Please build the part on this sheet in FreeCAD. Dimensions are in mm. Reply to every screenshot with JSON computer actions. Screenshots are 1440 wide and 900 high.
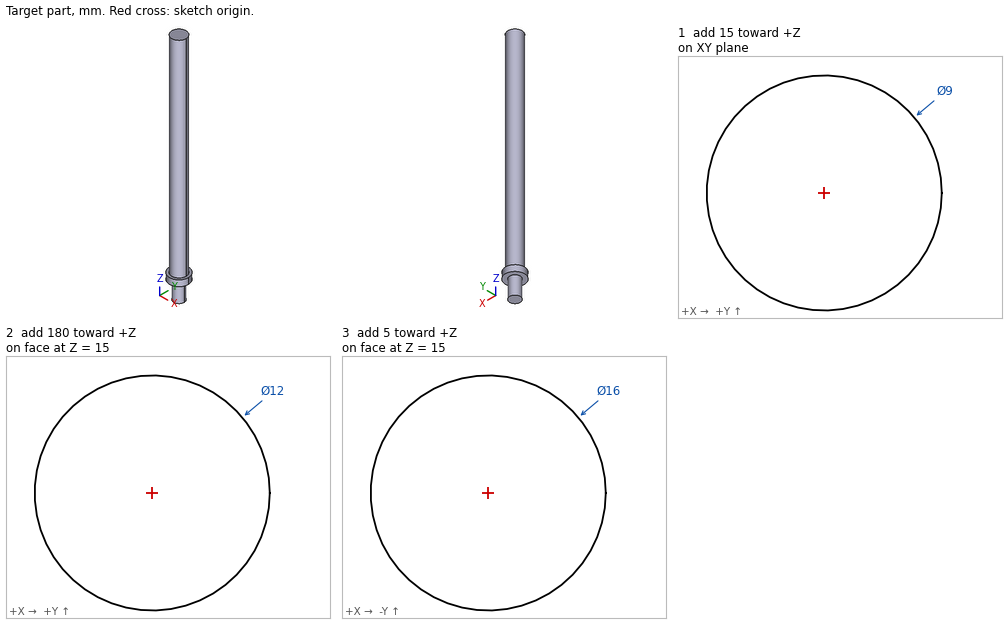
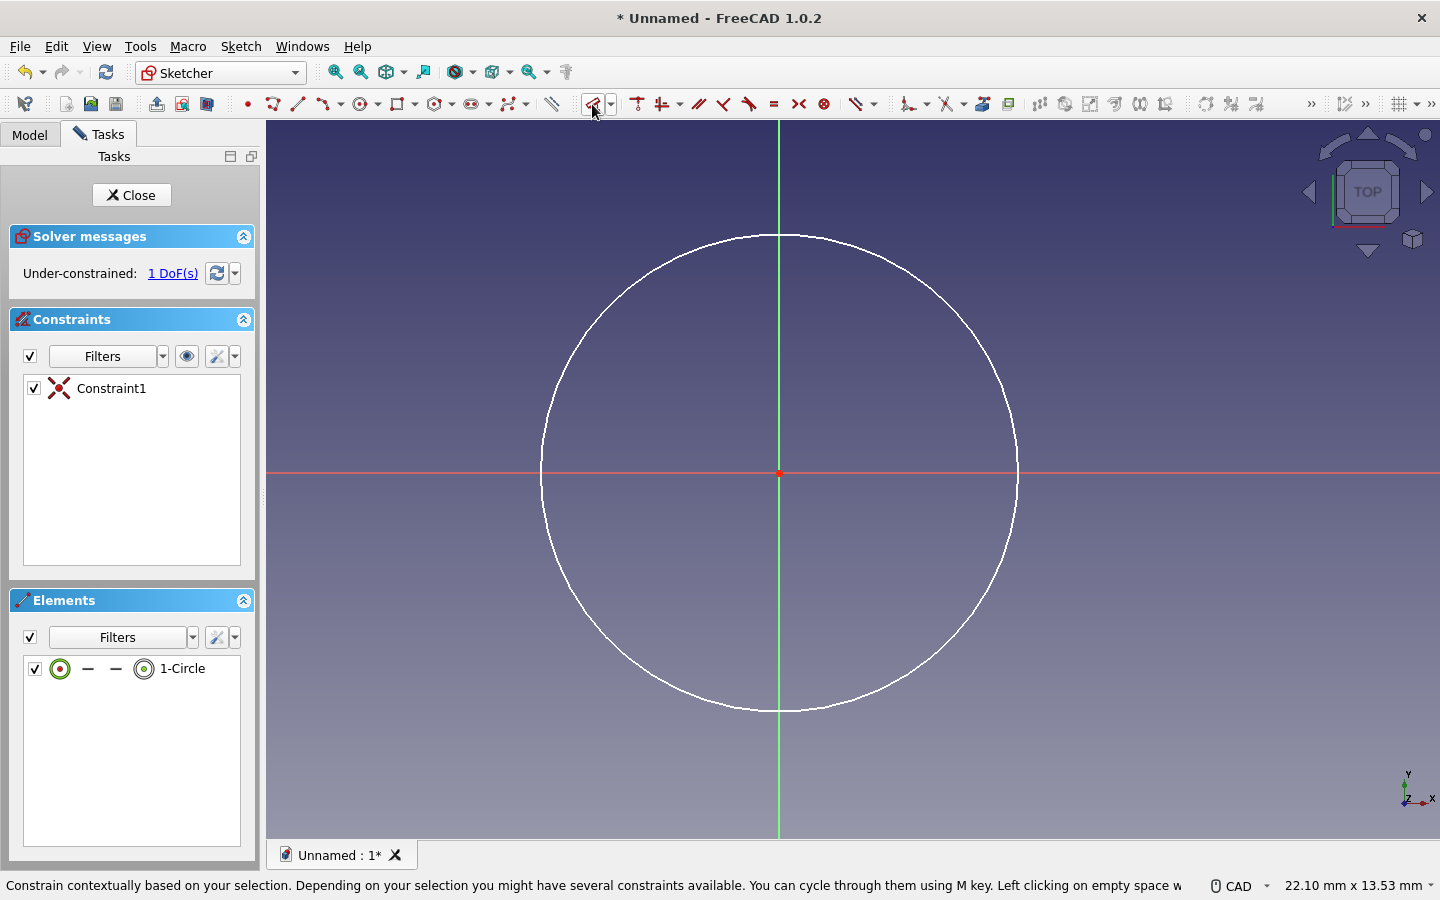
{"action": "left_click", "coordinate": [948, 304]}
{"action": "left_click", "coordinate": [971, 281]}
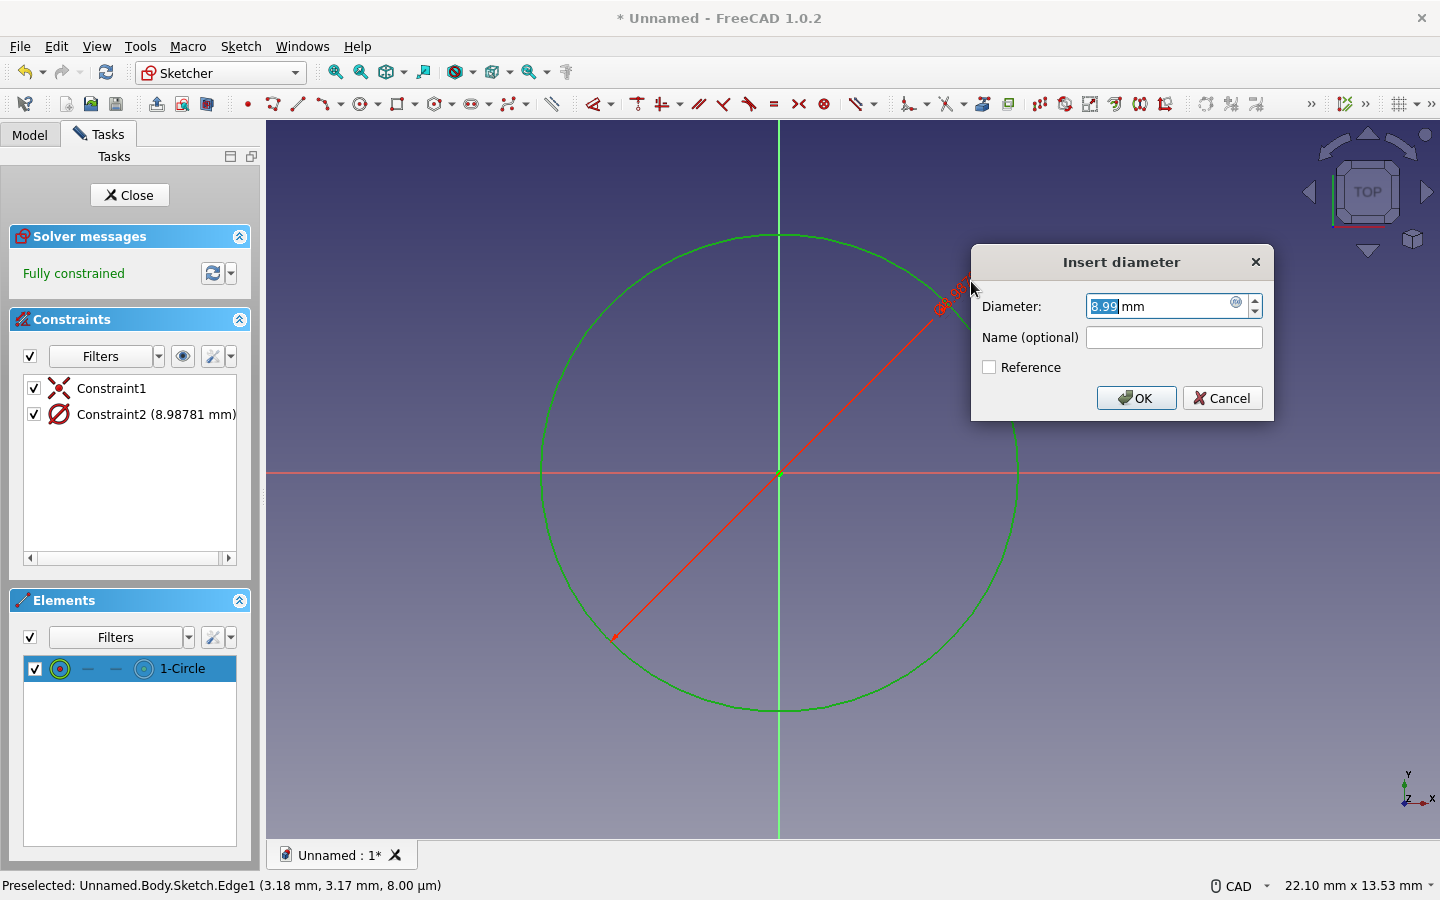
{"action": "type", "text": "9"}
{"action": "key", "text": "Return"}
{"action": "key", "text": "Escape"}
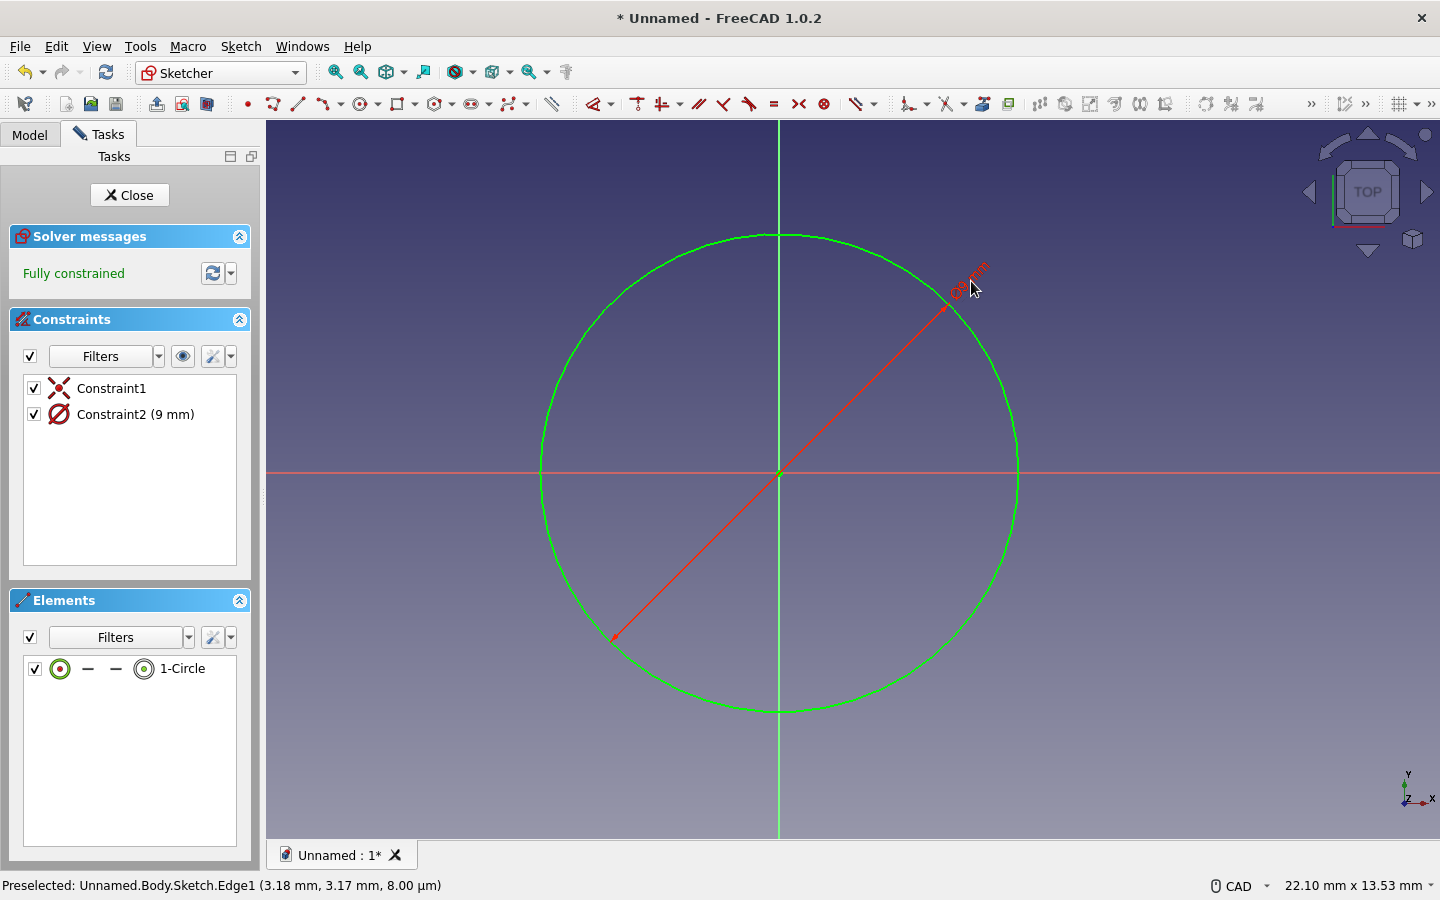
{"action": "left_click", "coordinate": [130, 195]}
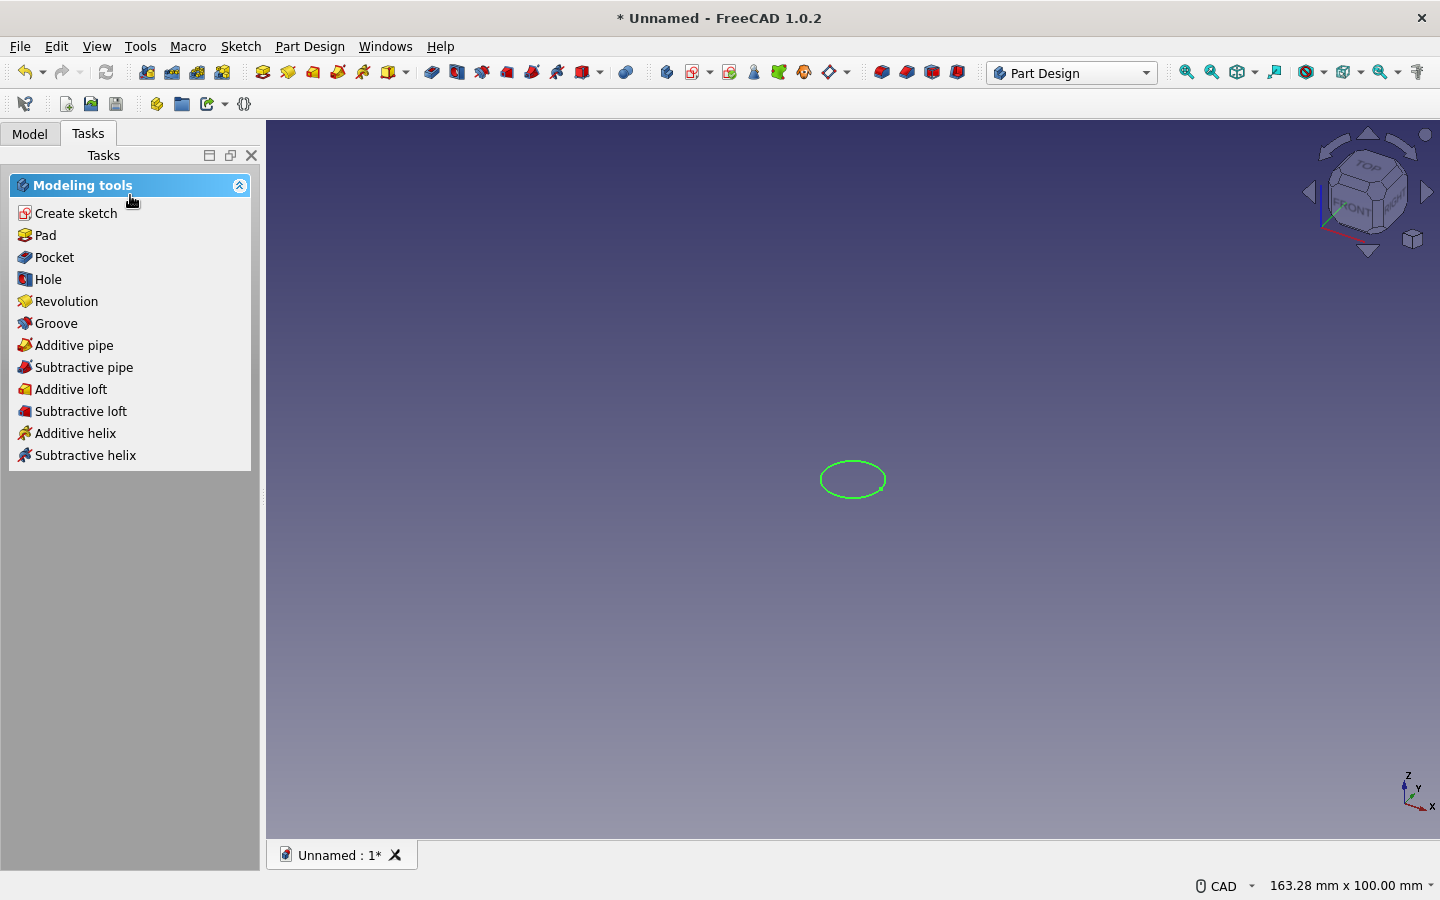
{"action": "left_click", "coordinate": [263, 72]}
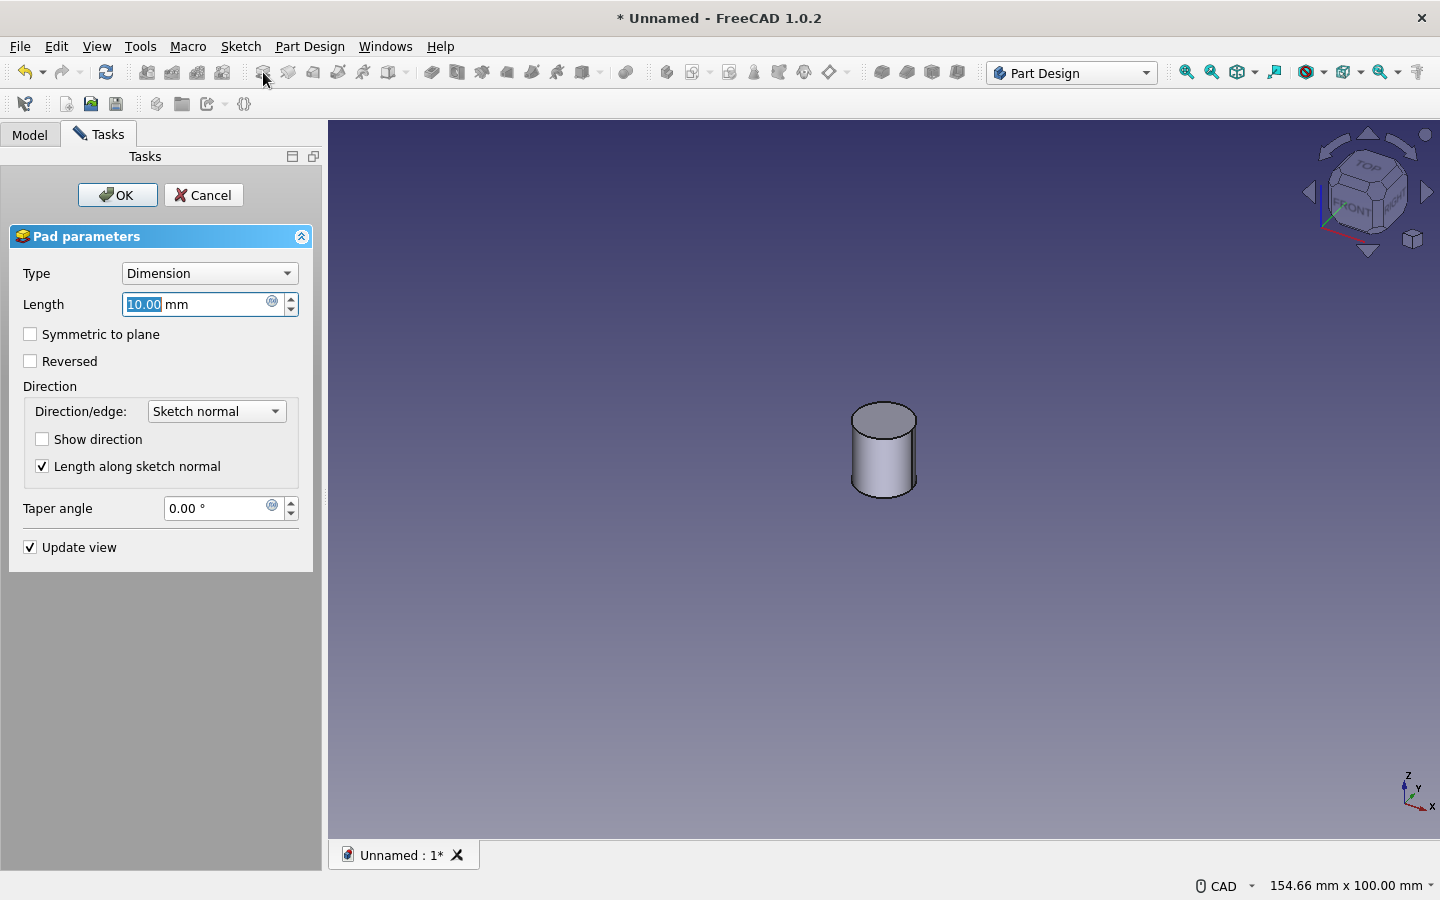
{"action": "type", "text": "15"}
{"action": "key", "text": "Tab"}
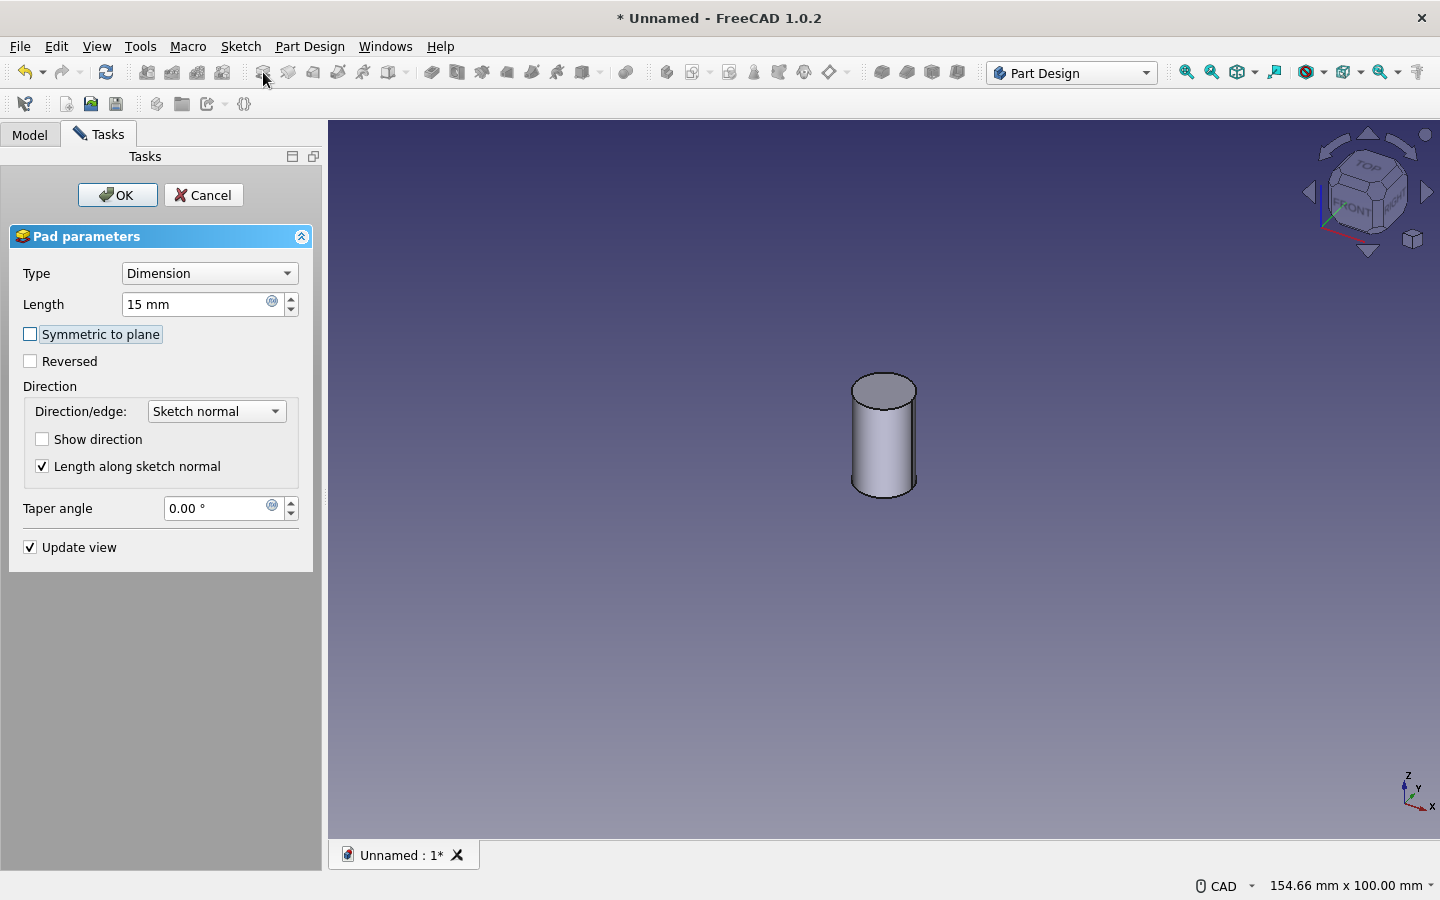
{"action": "left_click", "coordinate": [118, 195]}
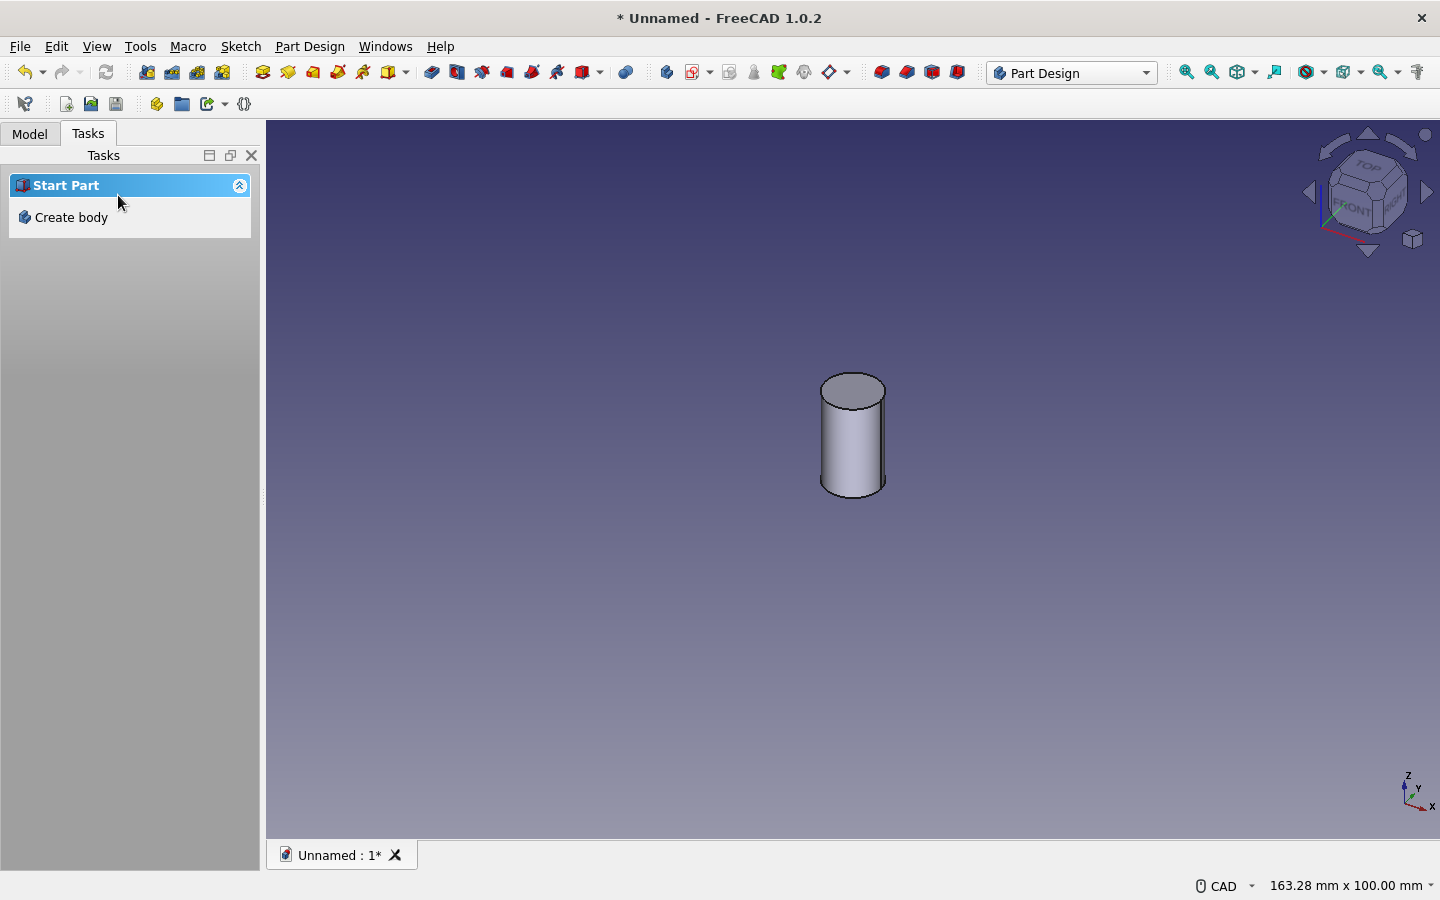
{"action": "key", "text": "v f"}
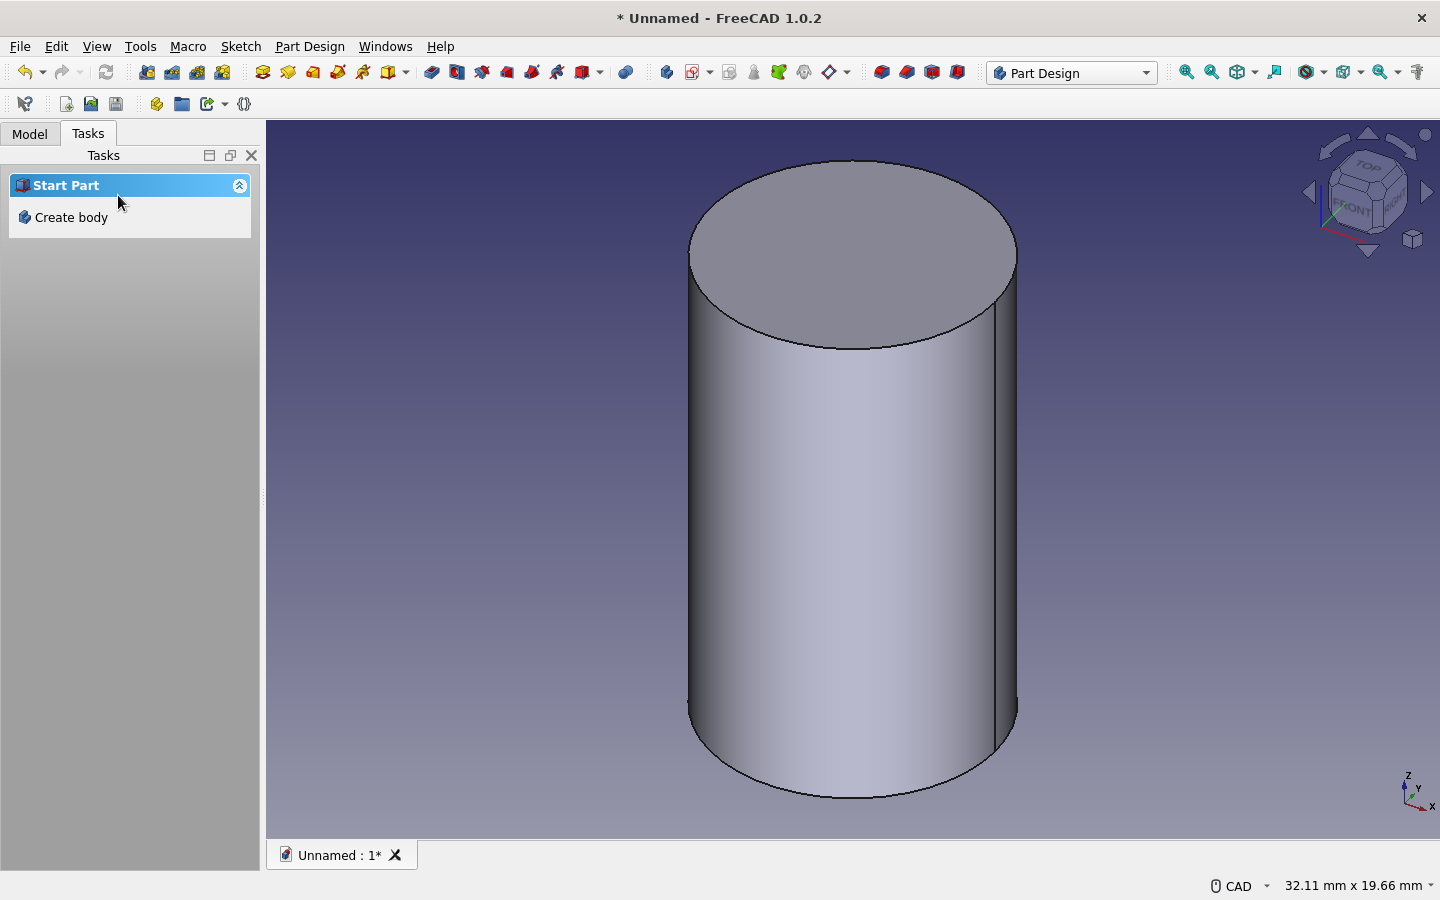
{"action": "left_click", "coordinate": [853, 254]}